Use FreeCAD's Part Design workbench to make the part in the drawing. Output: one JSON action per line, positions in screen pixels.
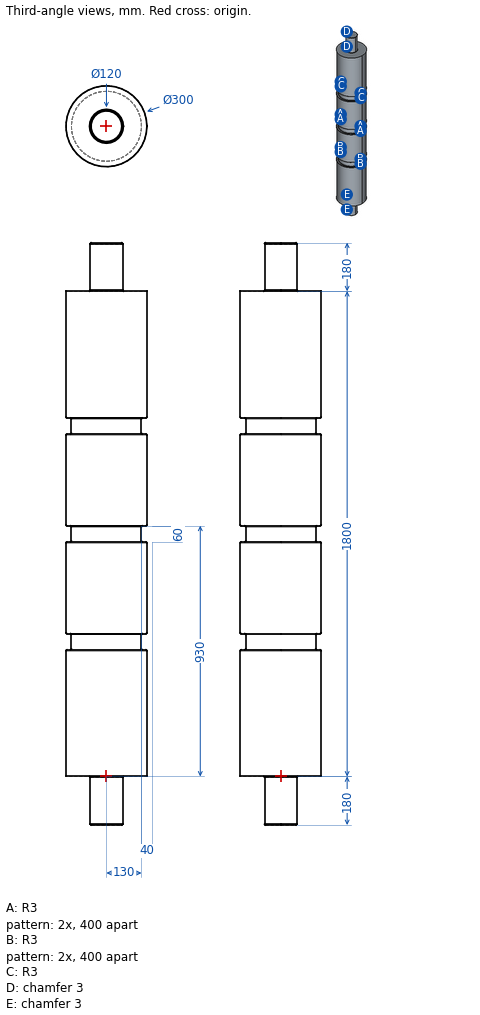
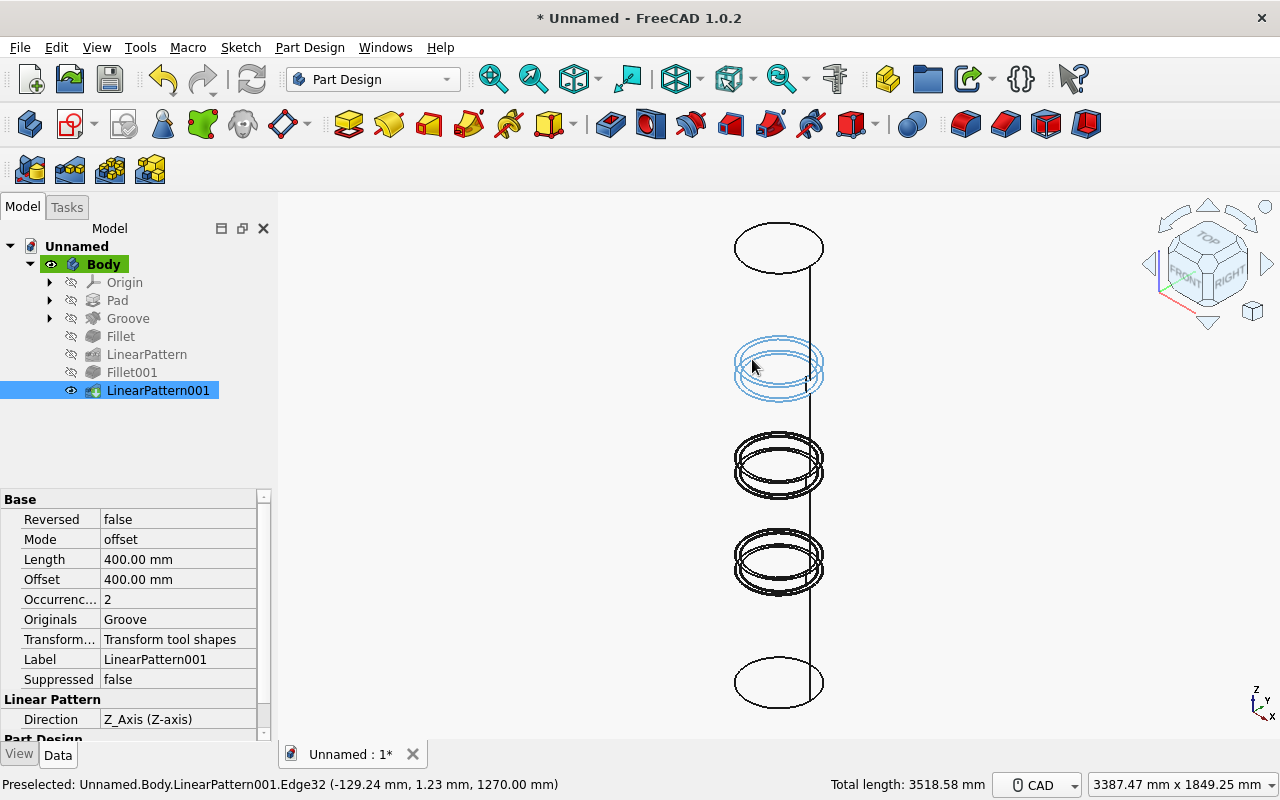
{"action": "key", "text": "v 1"}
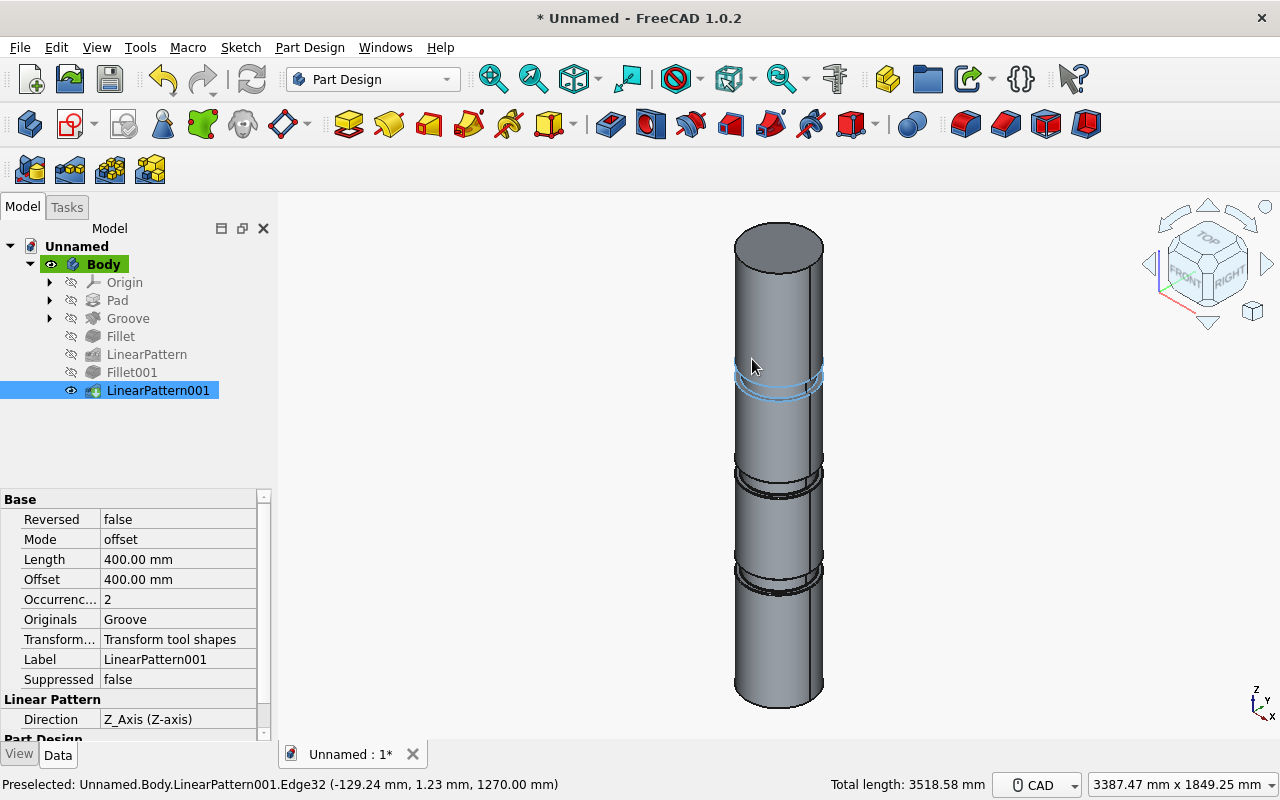
{"action": "left_click", "coordinate": [966, 124]}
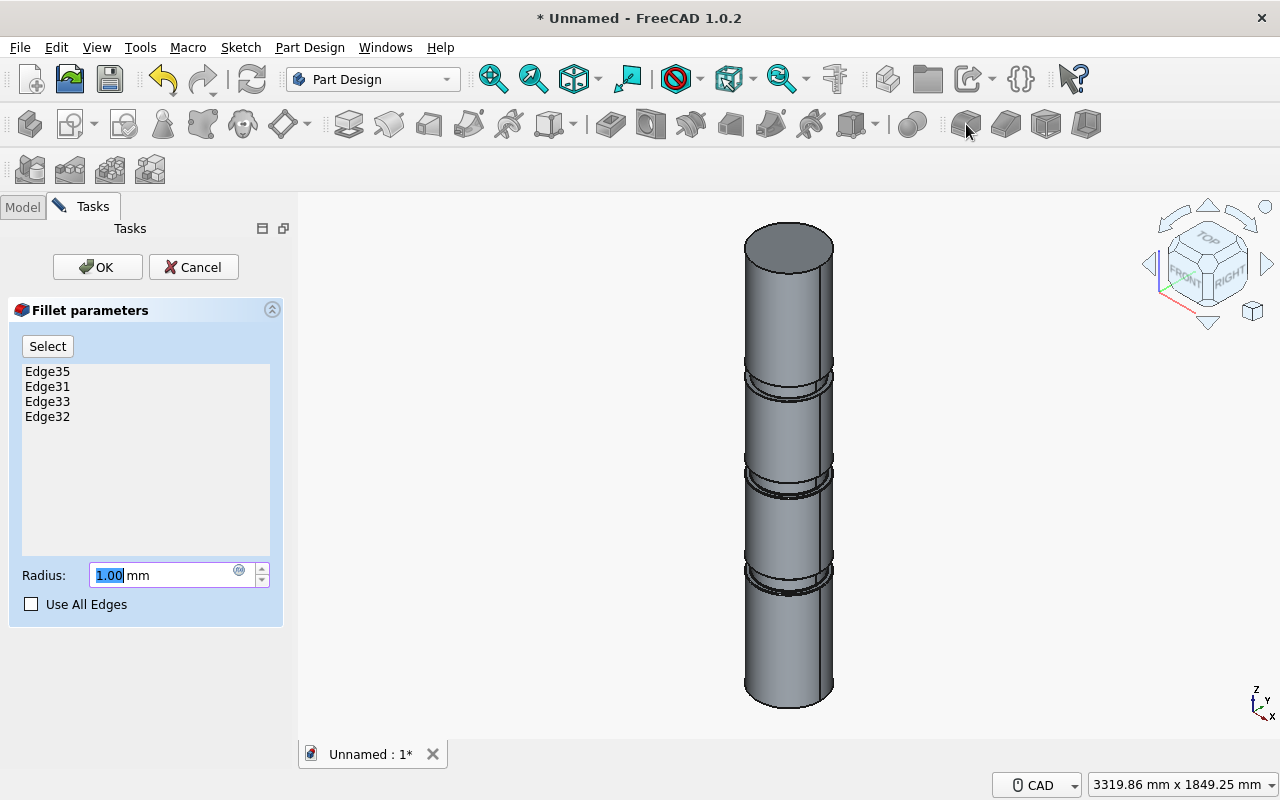
{"action": "type", "text": "3"}
{"action": "key", "text": "Tab"}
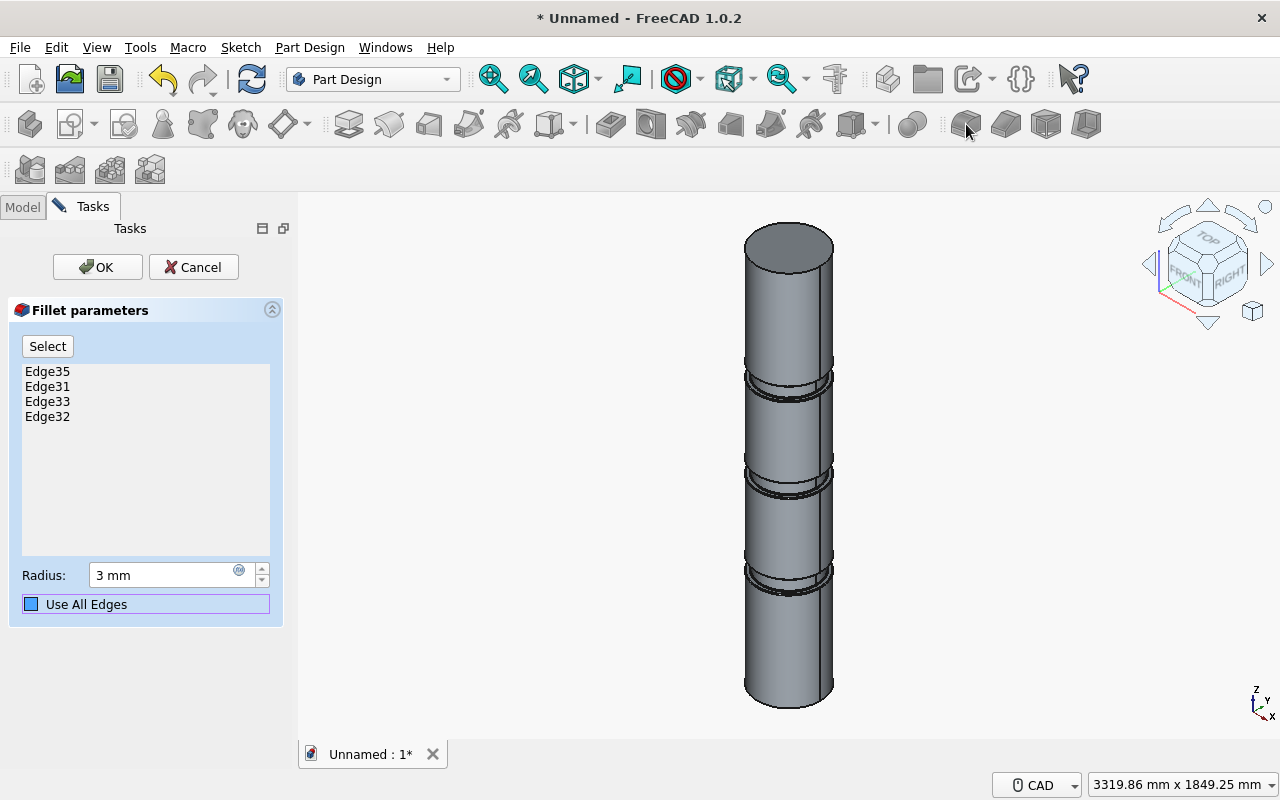
{"action": "left_click", "coordinate": [98, 267]}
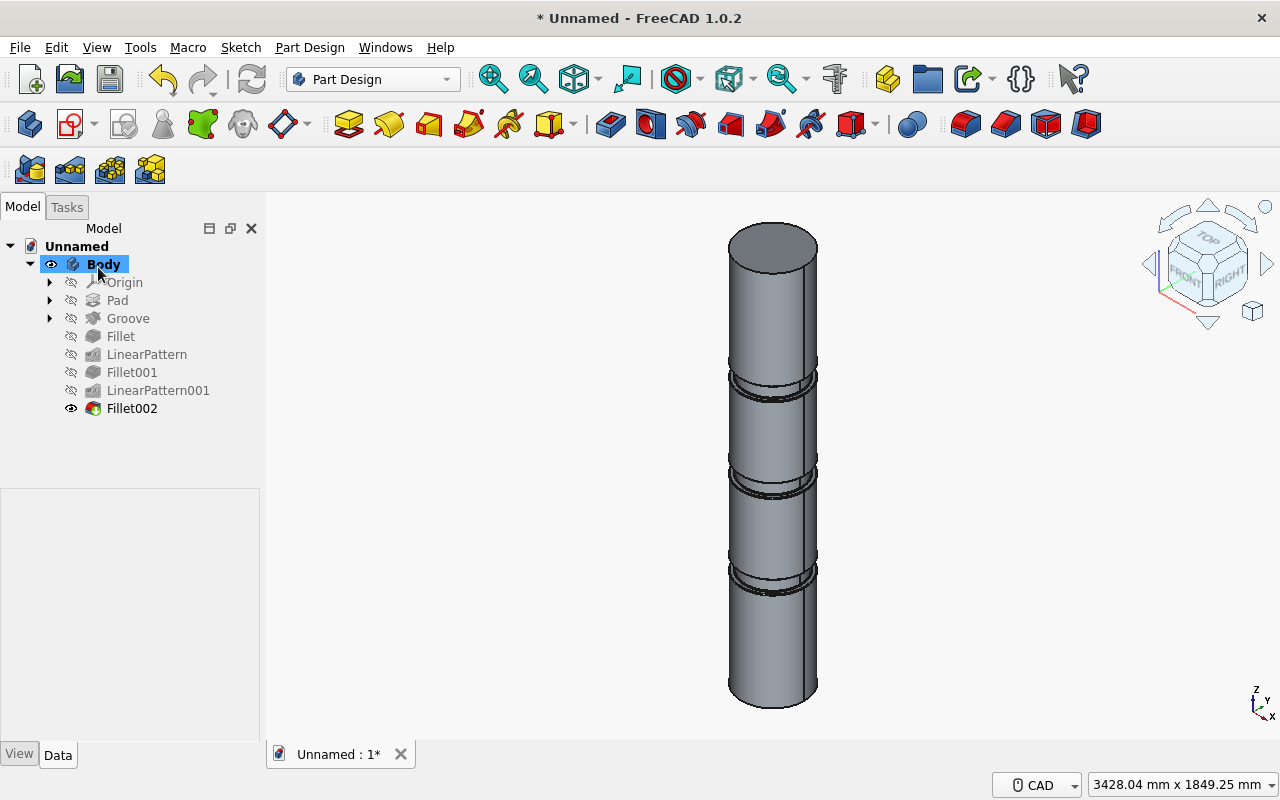
{"action": "left_click", "coordinate": [773, 247]}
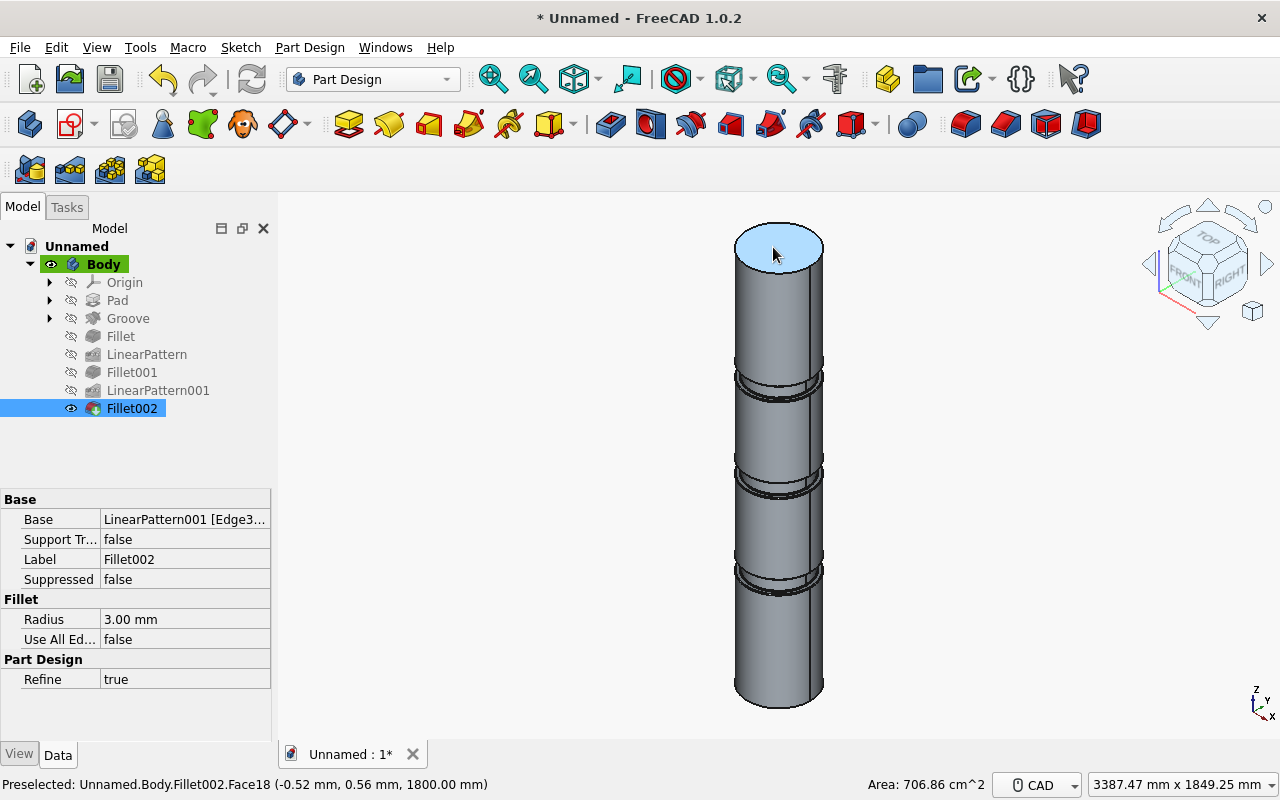
{"action": "left_click", "coordinate": [70, 124]}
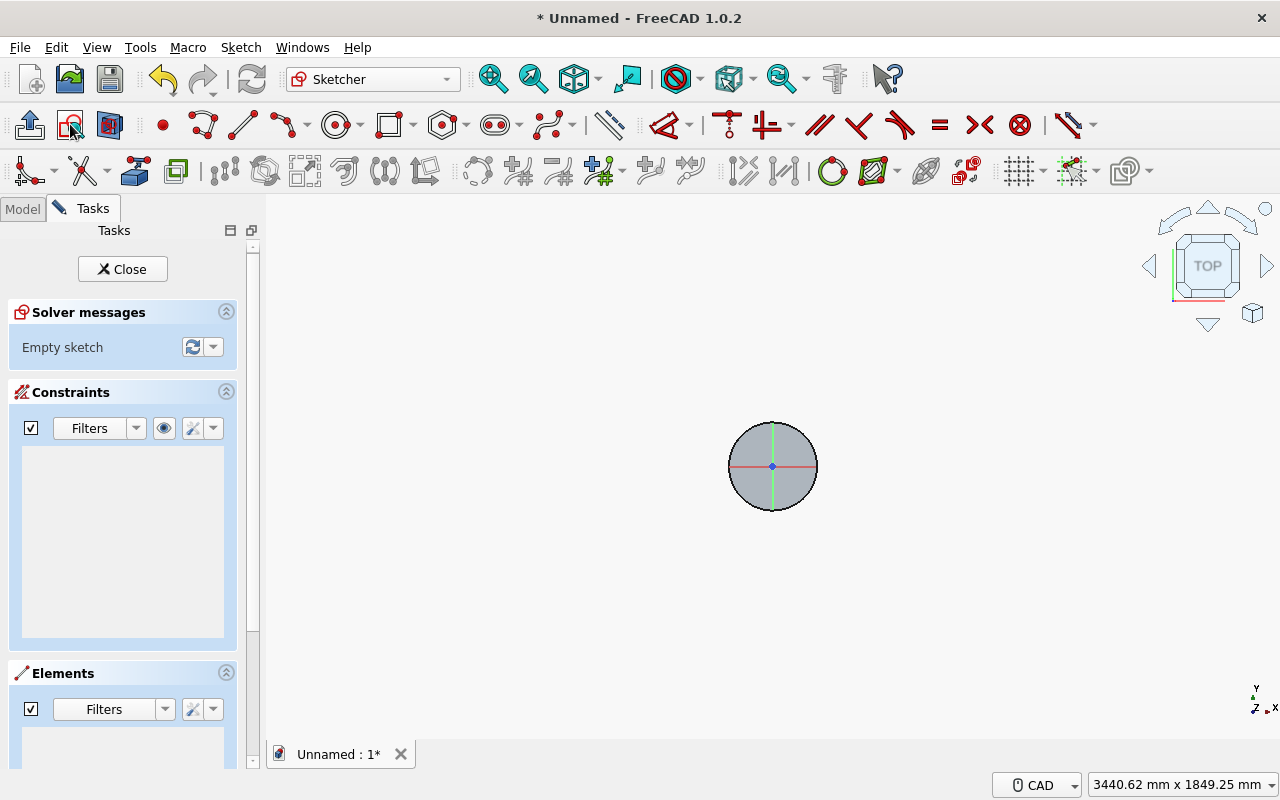
{"action": "scroll", "coordinate": [782, 467], "scroll_direction": "up", "scroll_amount": 11}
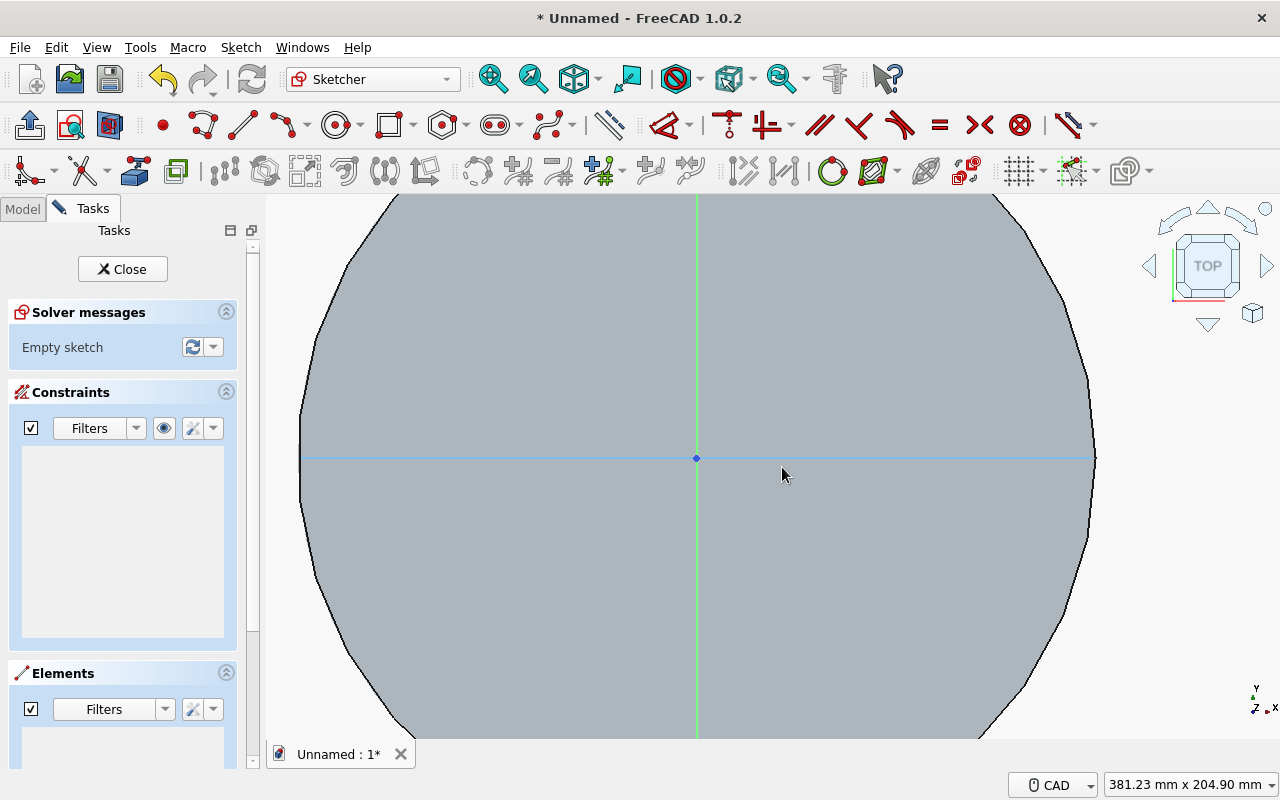
{"action": "left_click", "coordinate": [336, 126]}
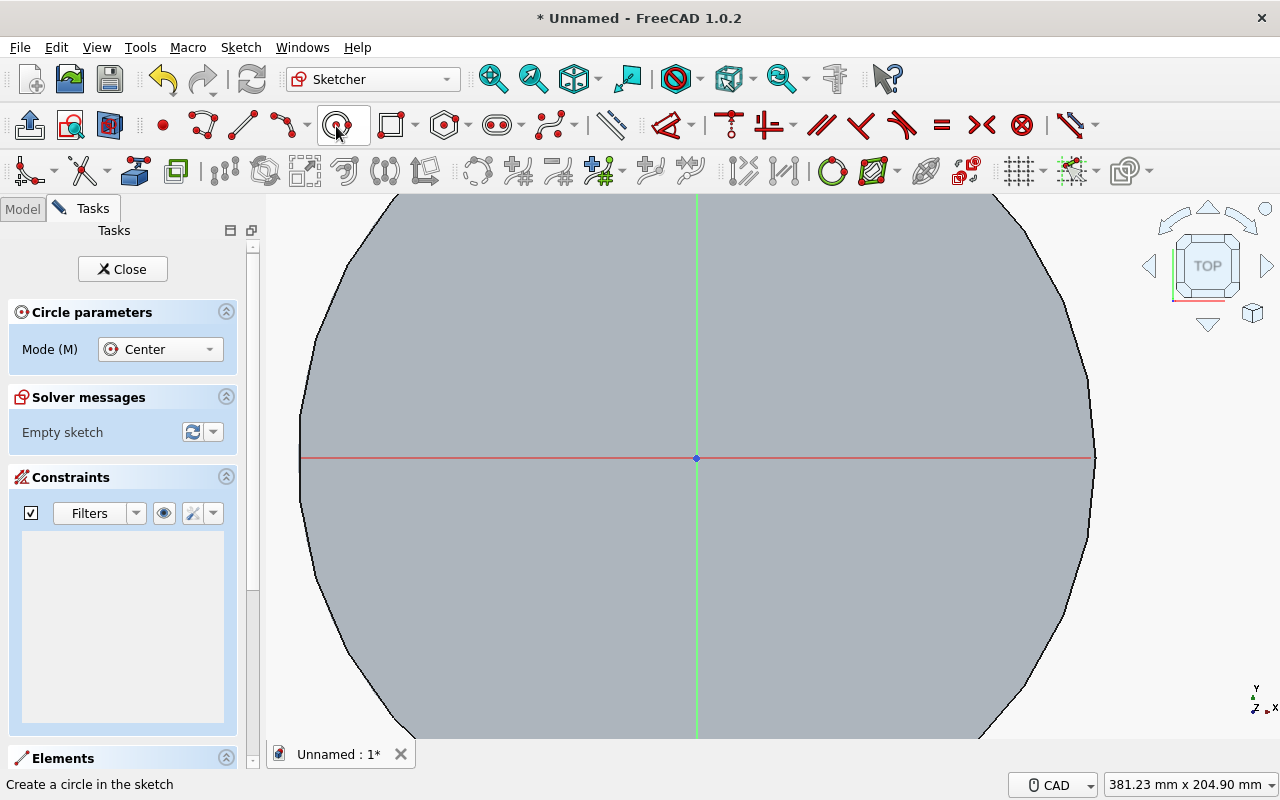
{"action": "left_click", "coordinate": [697, 458]}
{"action": "mouse_move", "coordinate": [809, 346]}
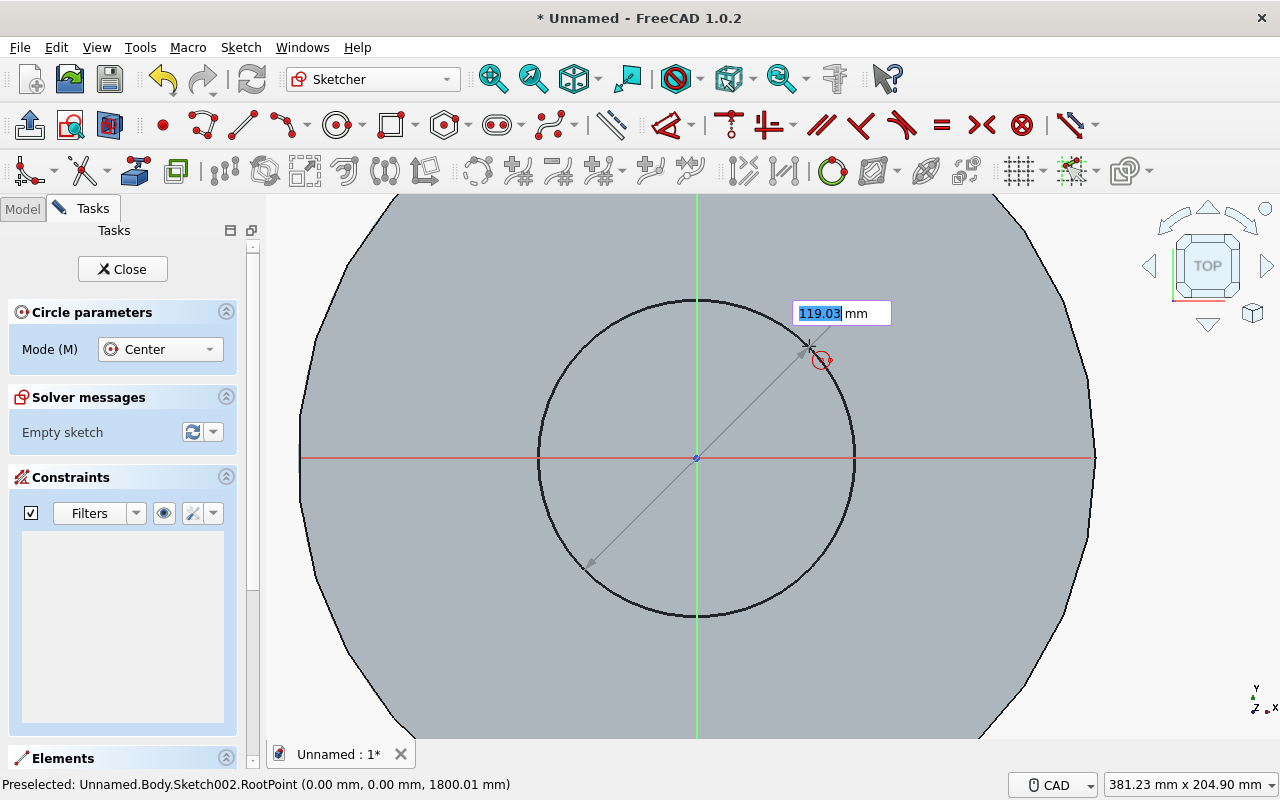
{"action": "type", "text": "120"}
{"action": "key", "text": "Return"}
{"action": "key", "text": "Escape"}